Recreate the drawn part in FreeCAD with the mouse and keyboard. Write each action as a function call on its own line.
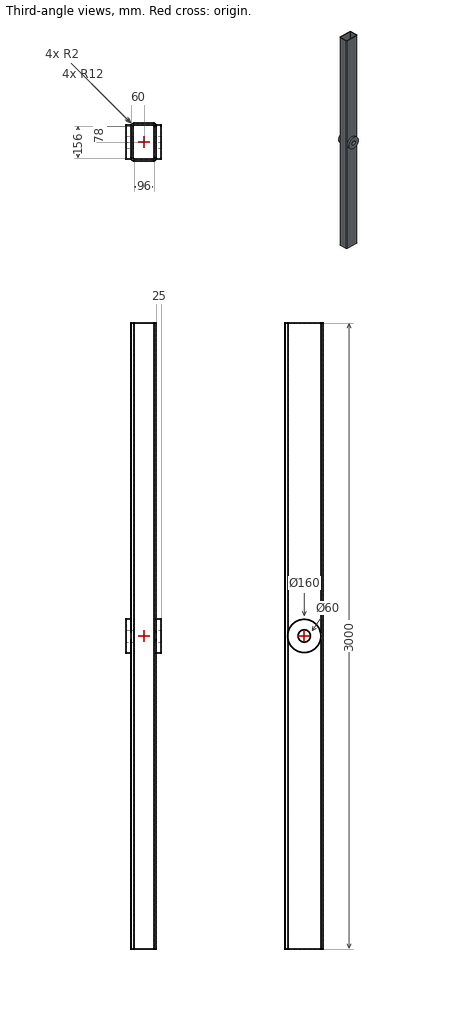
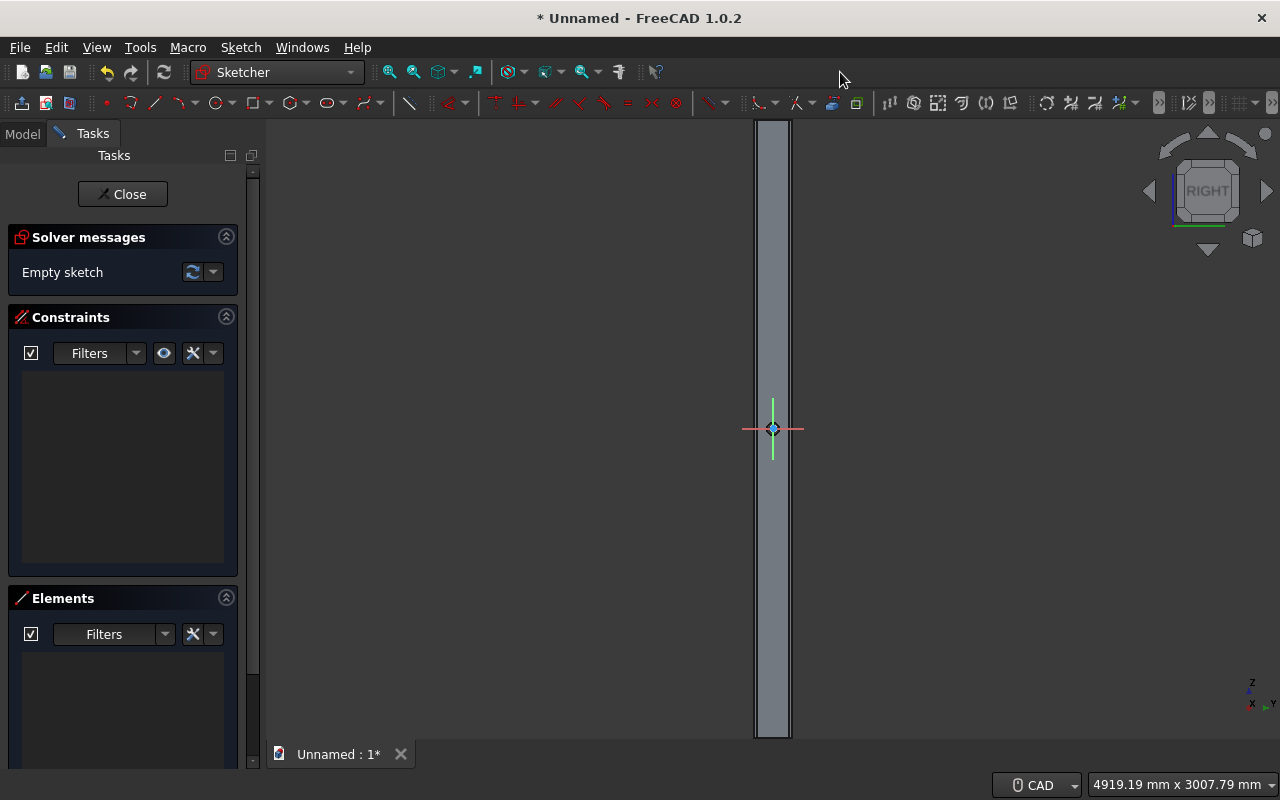
scroll(780, 429, up, 12)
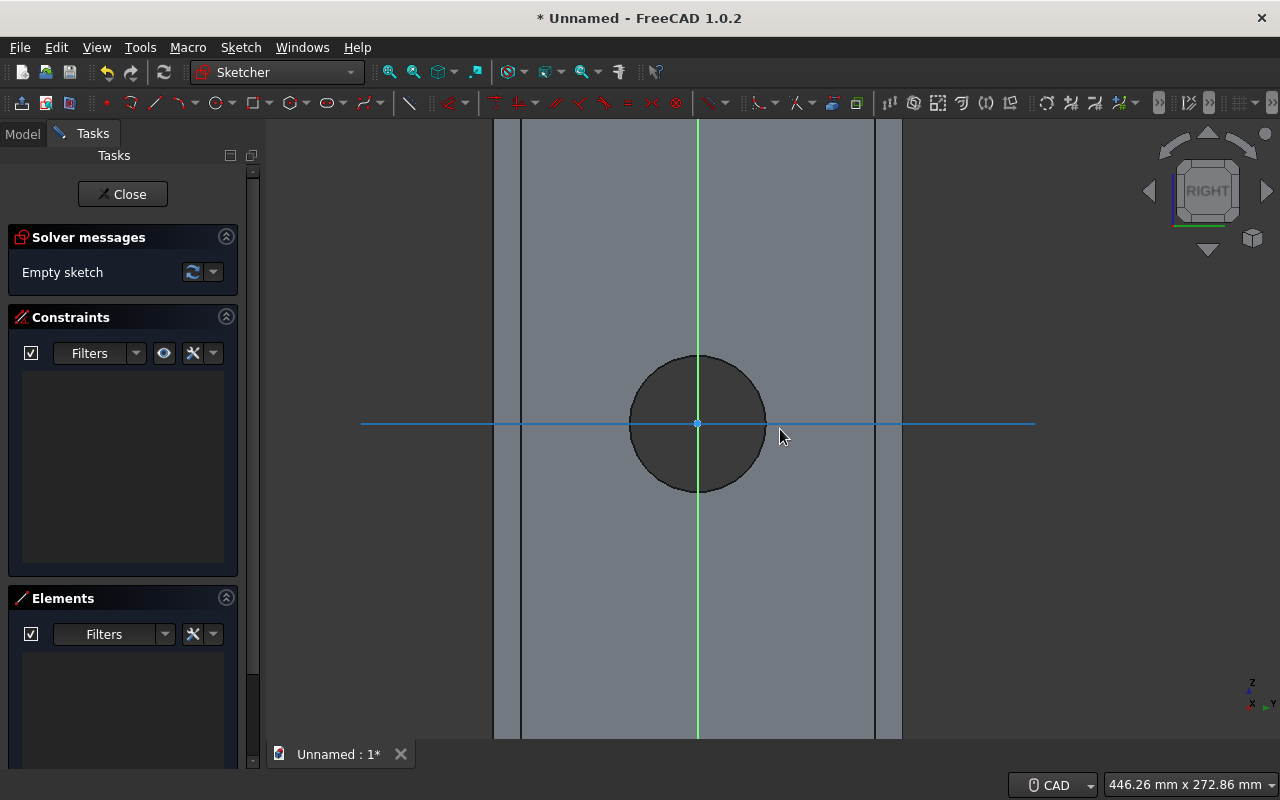
click(216, 104)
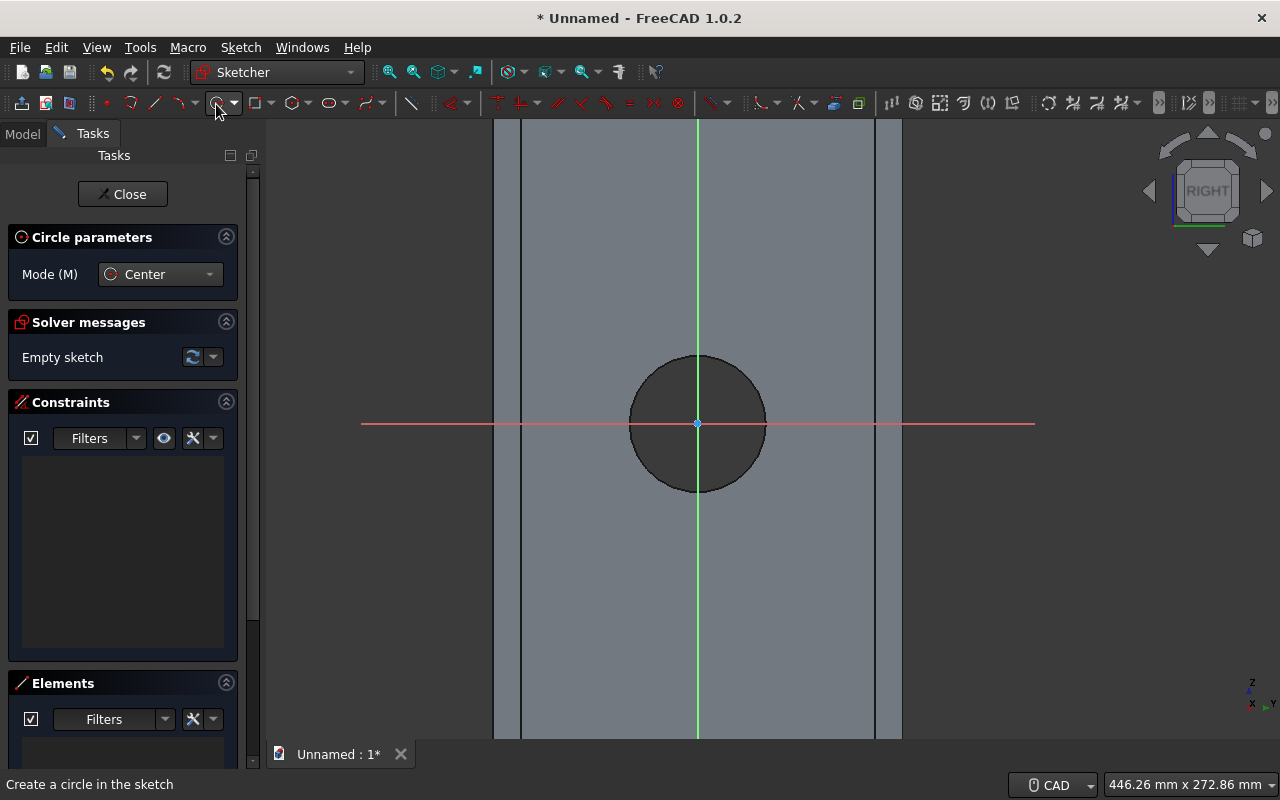
click(698, 424)
click(826, 295)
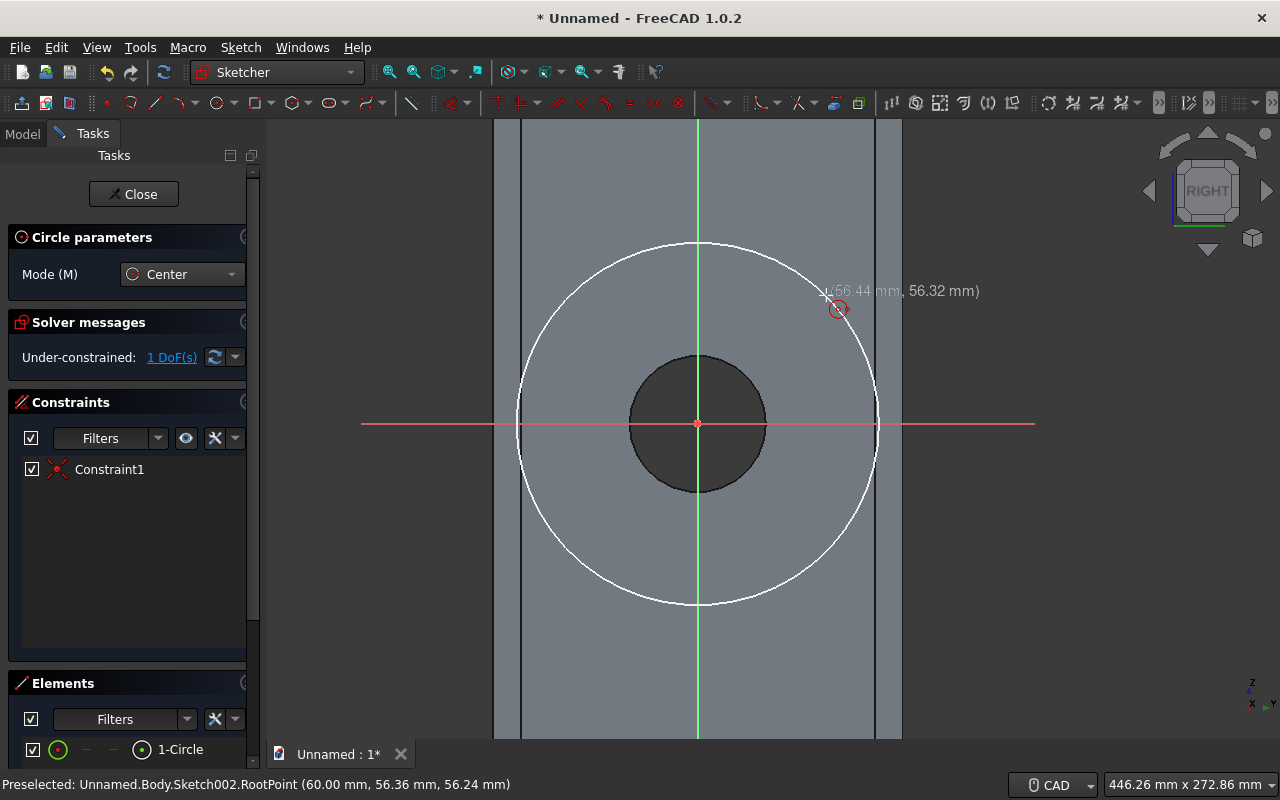
click(698, 424)
click(746, 376)
key(Escape)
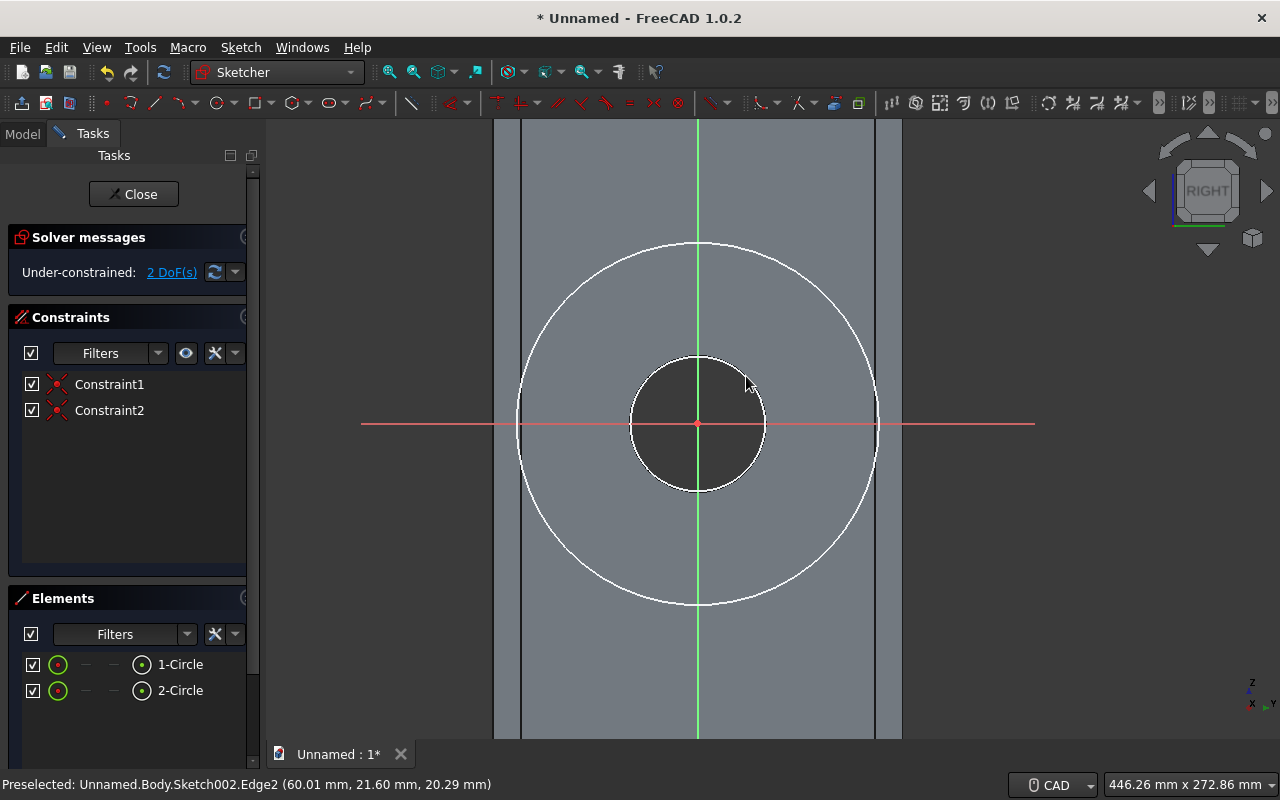
click(450, 104)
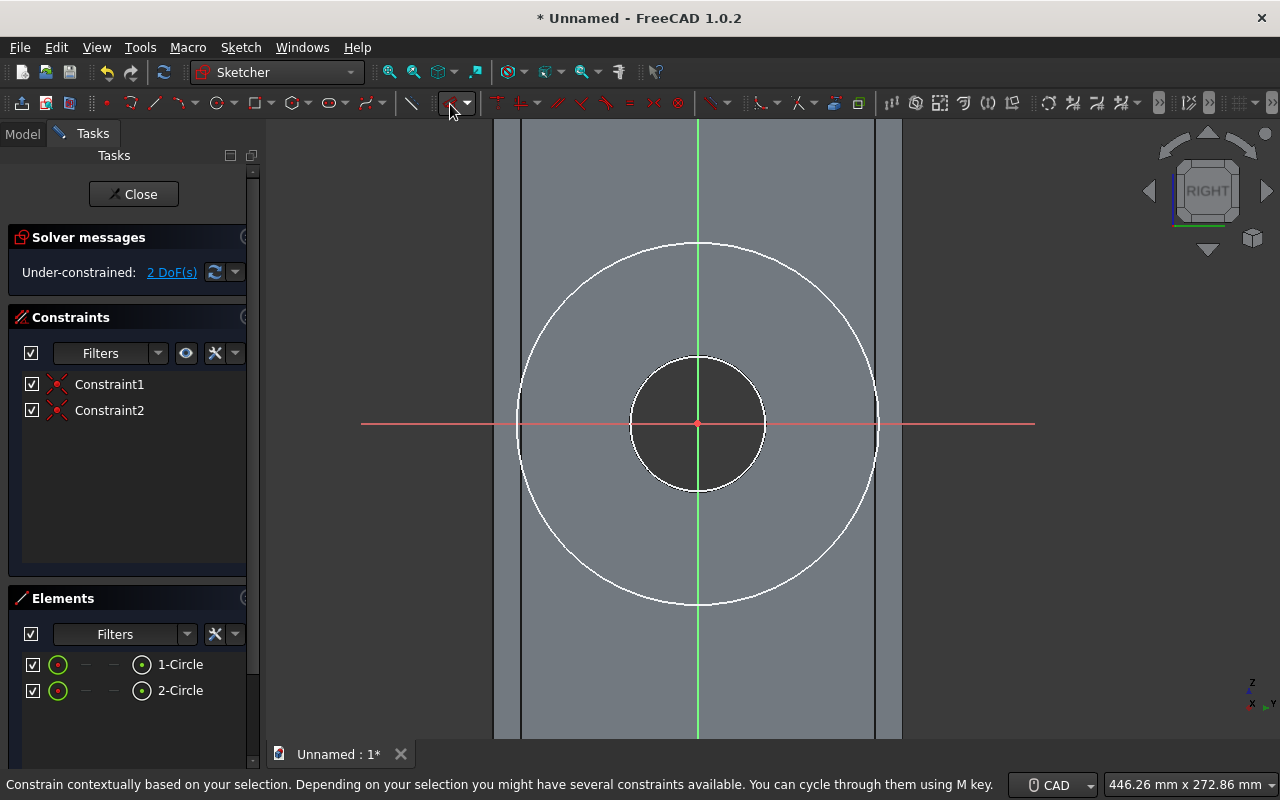
click(825, 295)
click(847, 272)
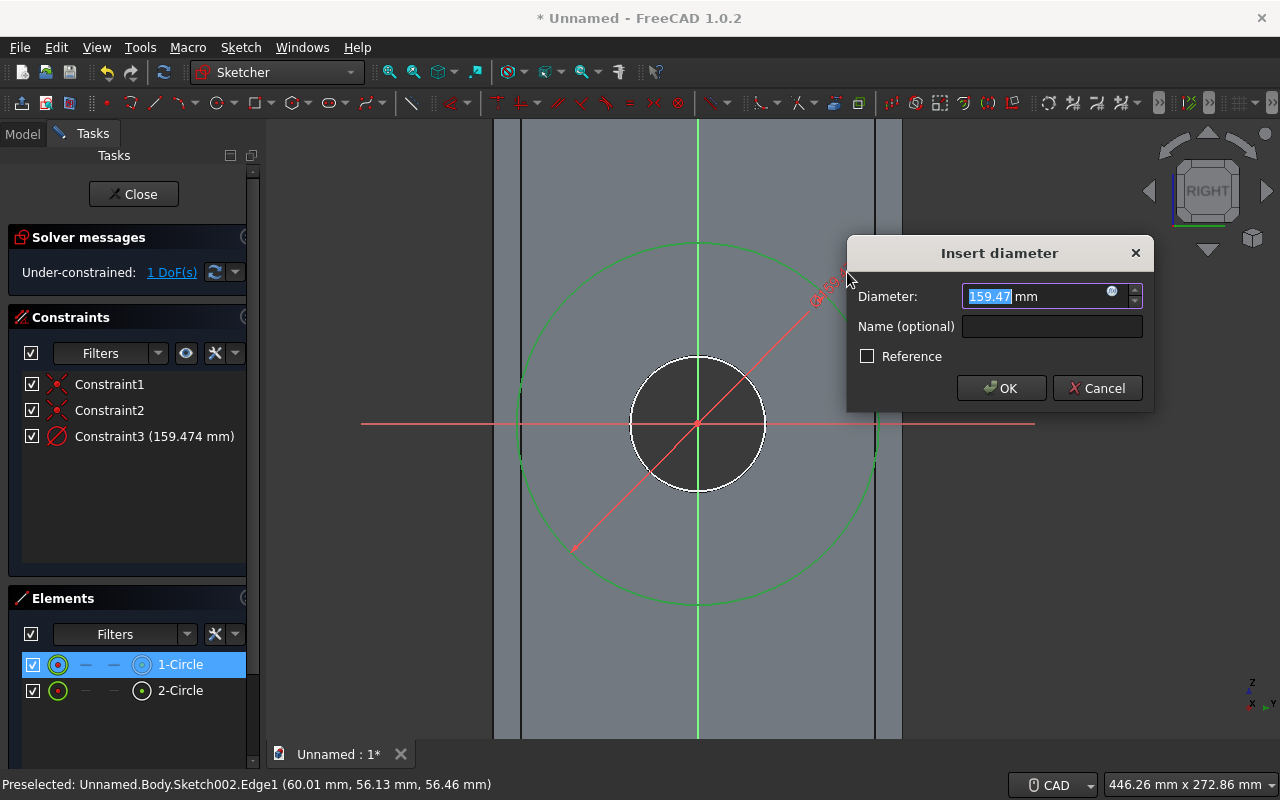
text(160)
key(Return)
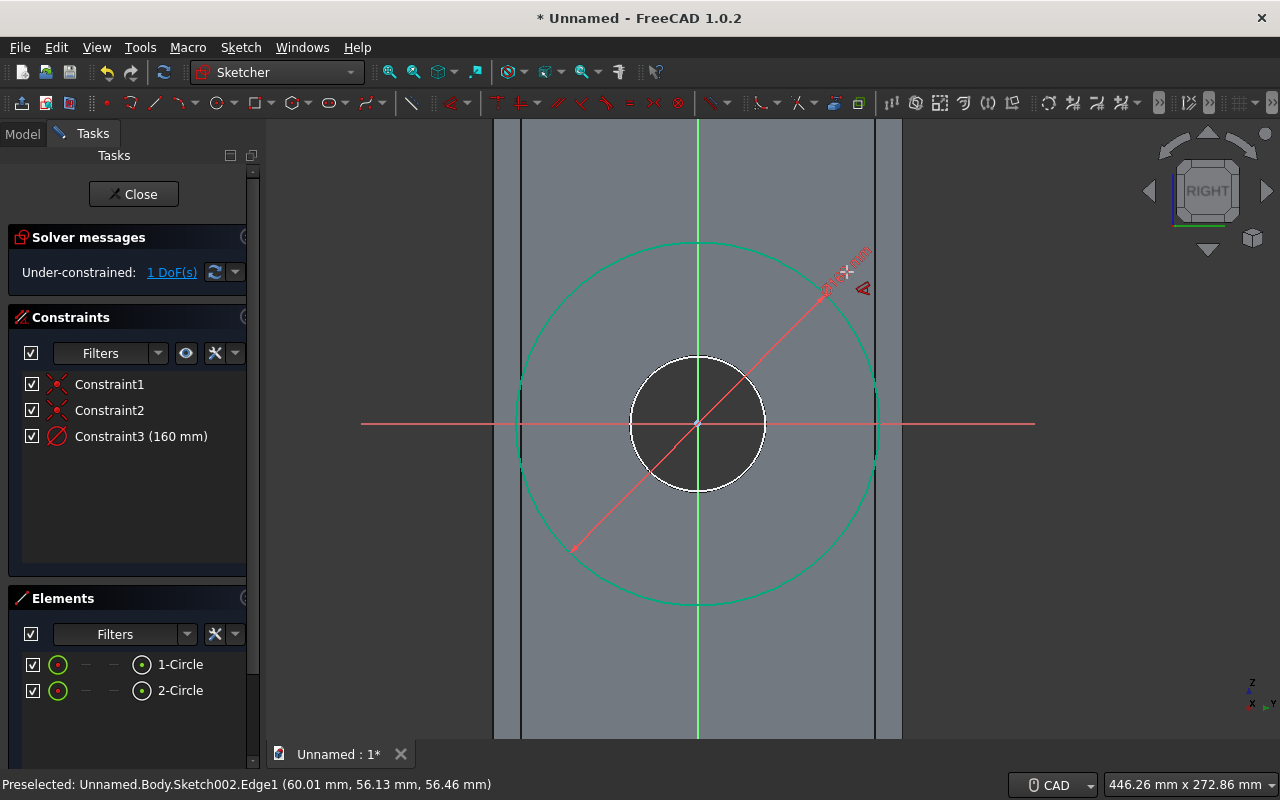
click(745, 376)
click(767, 353)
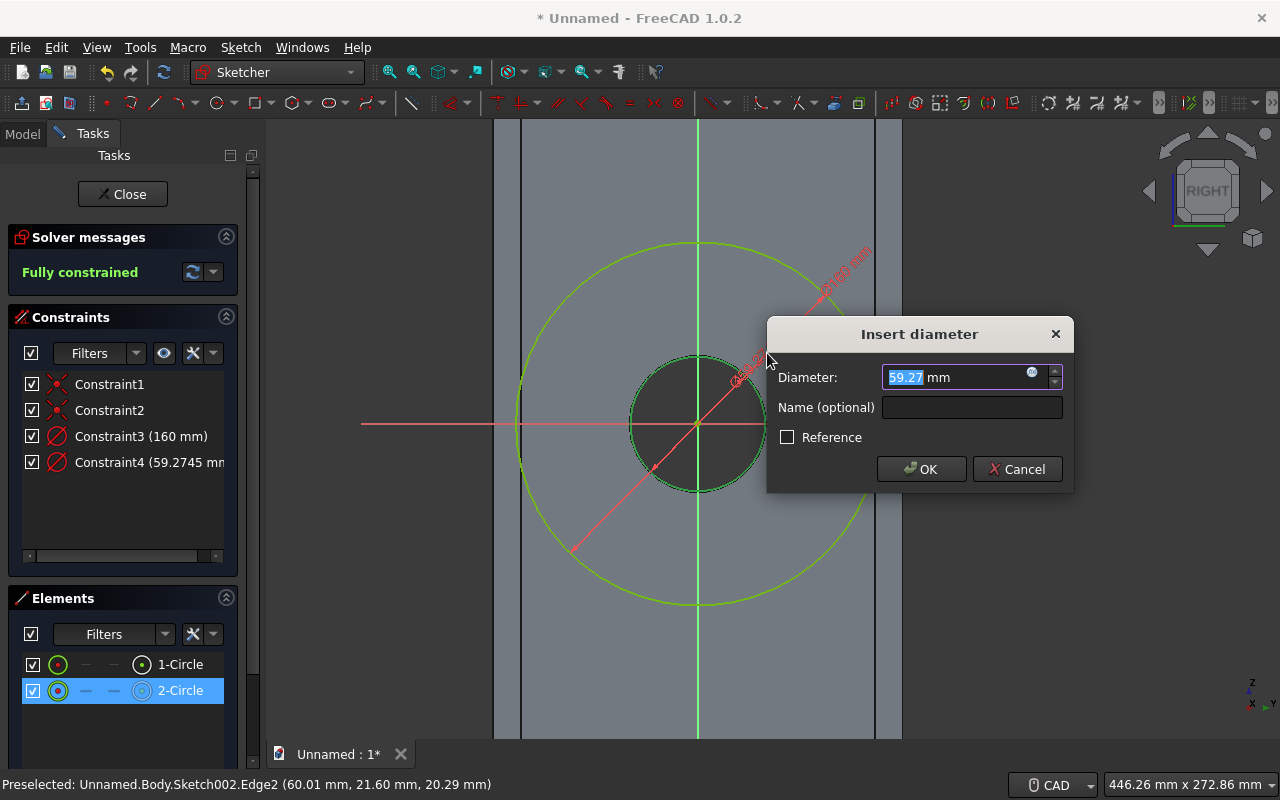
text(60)
key(Return)
key(Escape)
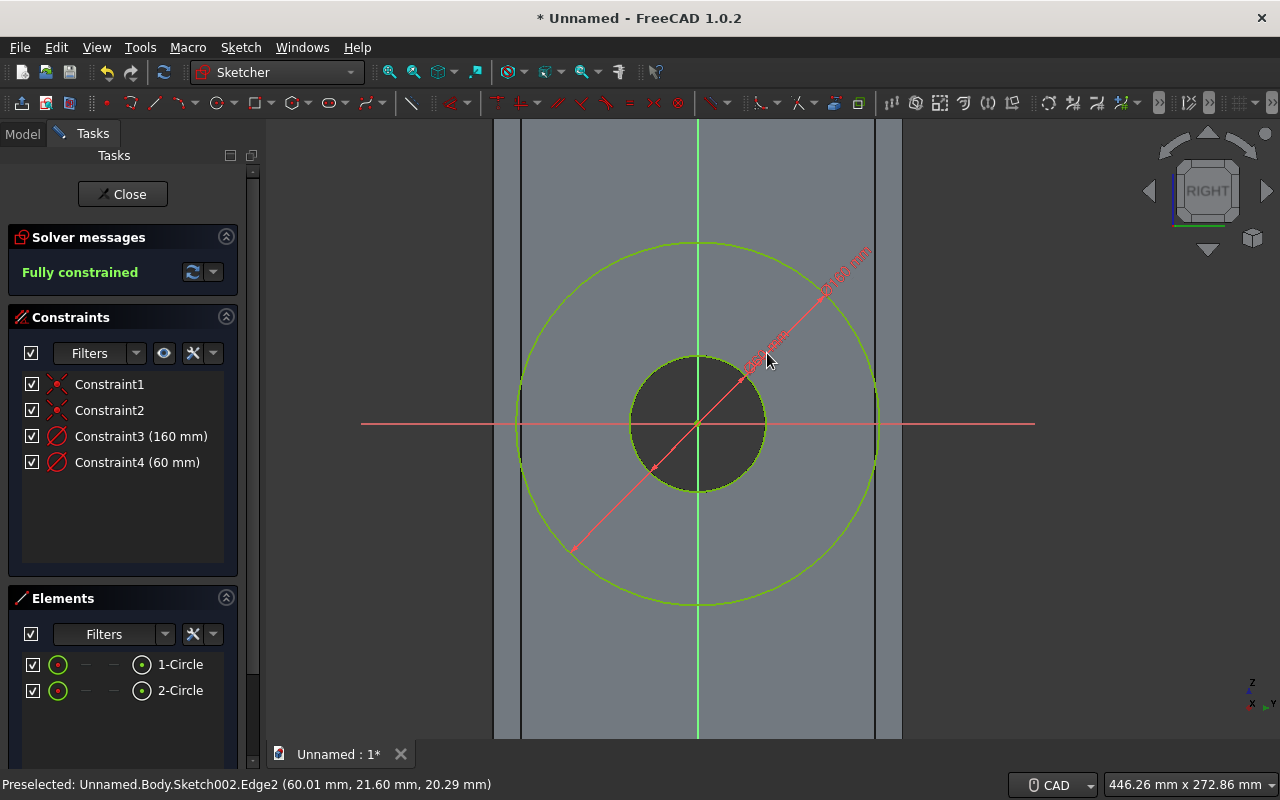
click(123, 194)